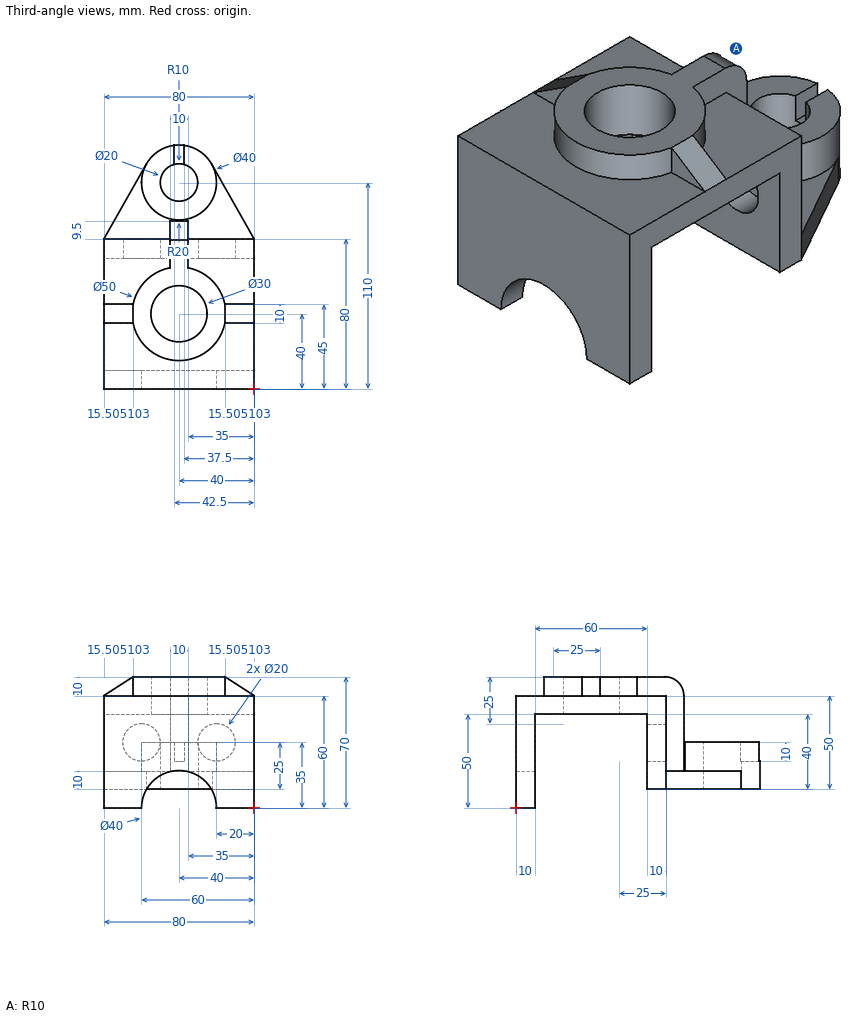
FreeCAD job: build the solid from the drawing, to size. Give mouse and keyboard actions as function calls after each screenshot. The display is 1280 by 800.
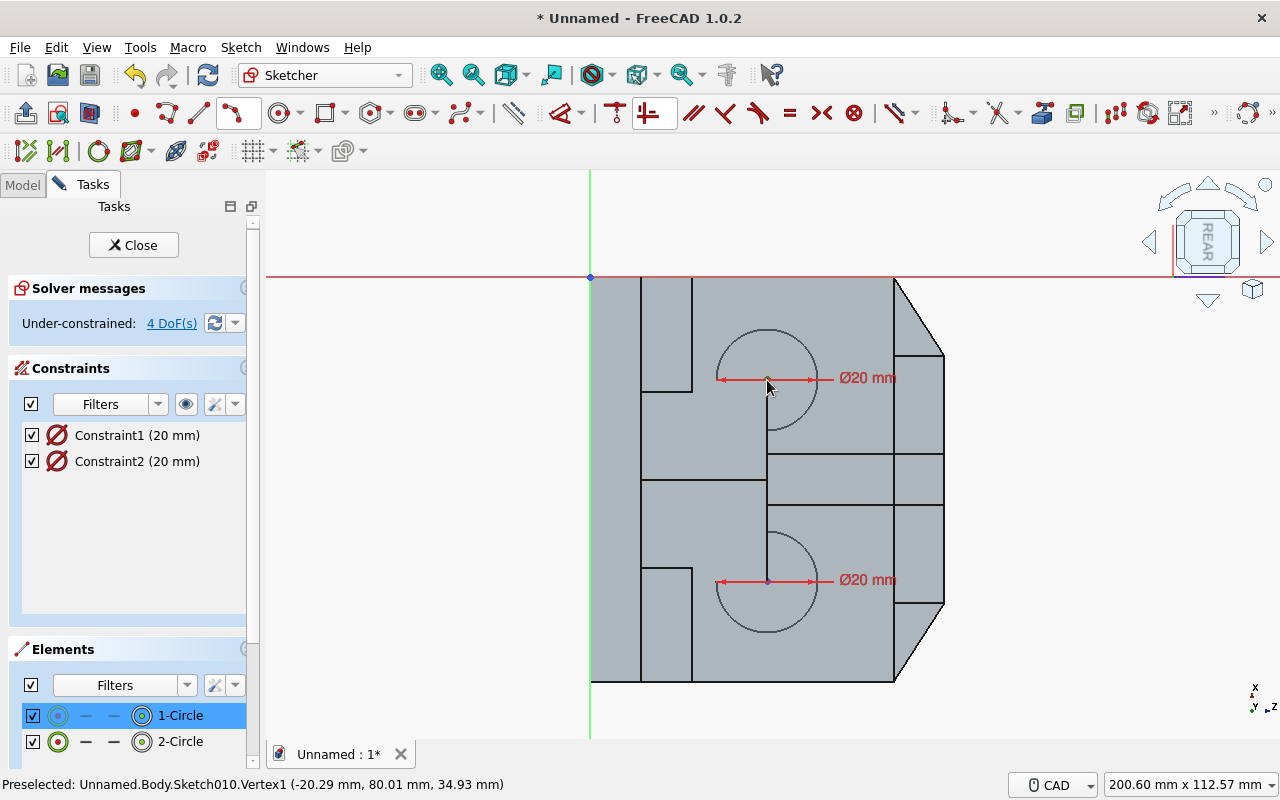
click(767, 582)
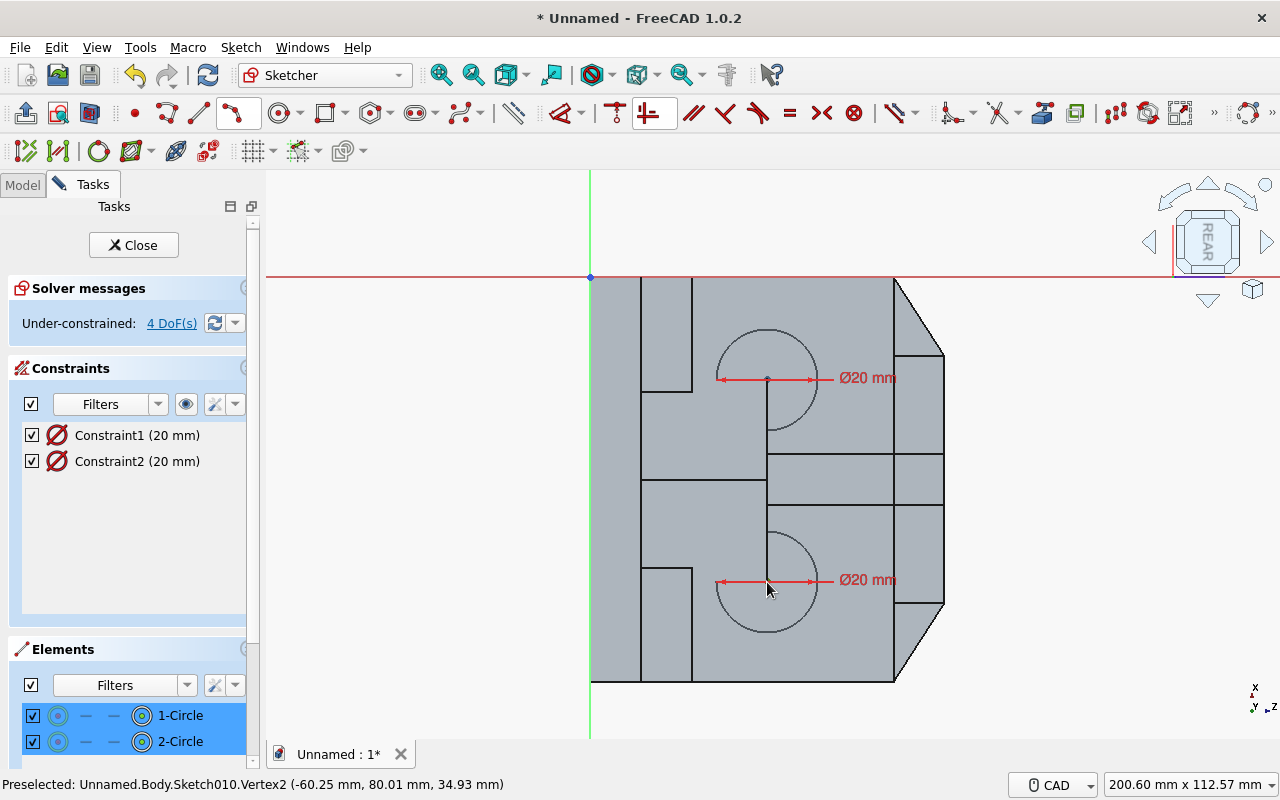
key(v)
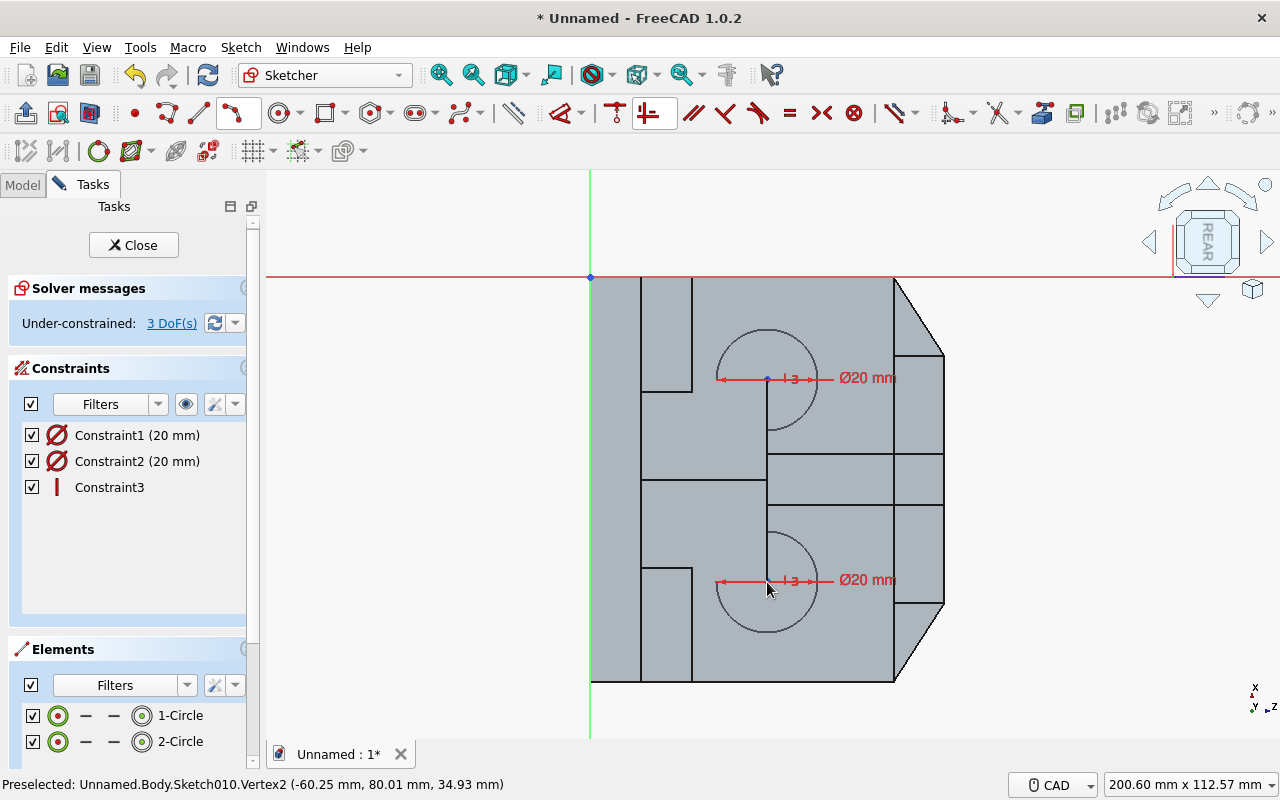
click(560, 114)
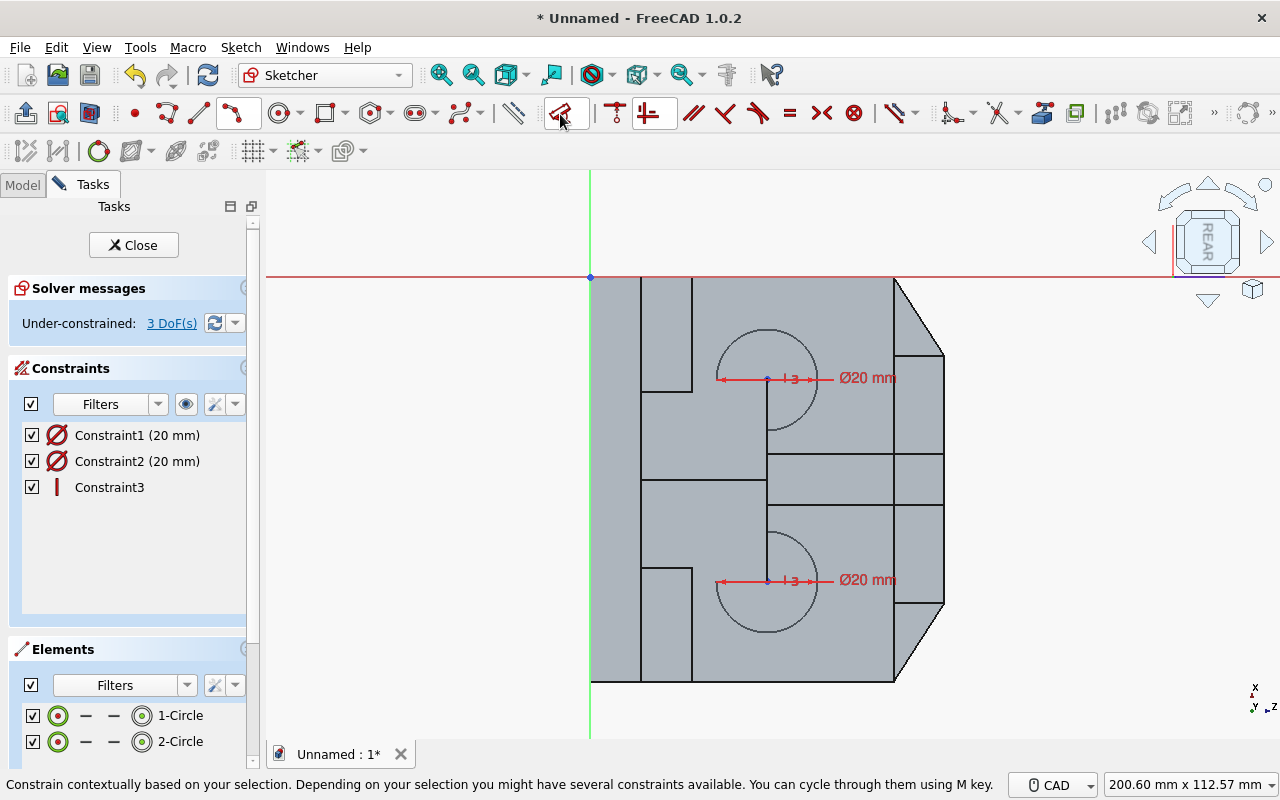
click(767, 380)
click(679, 243)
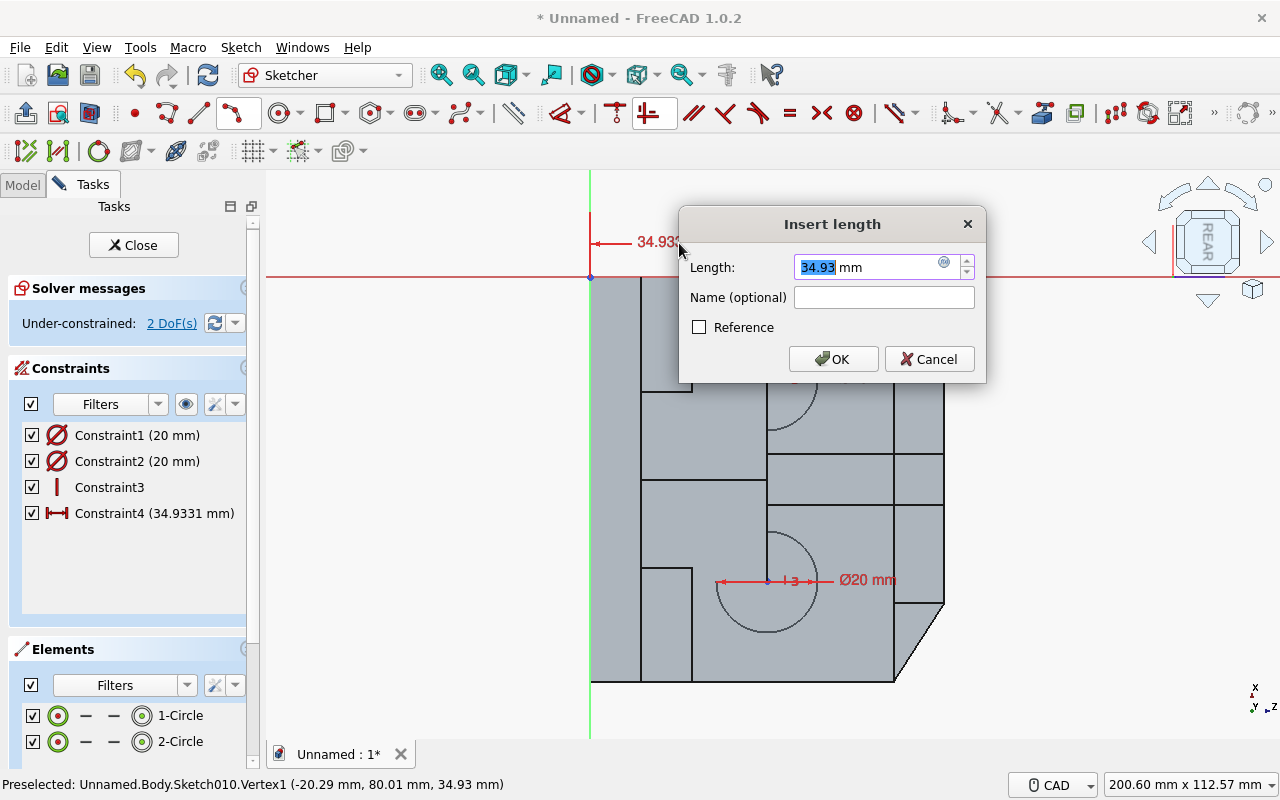
text(35)
key(Return)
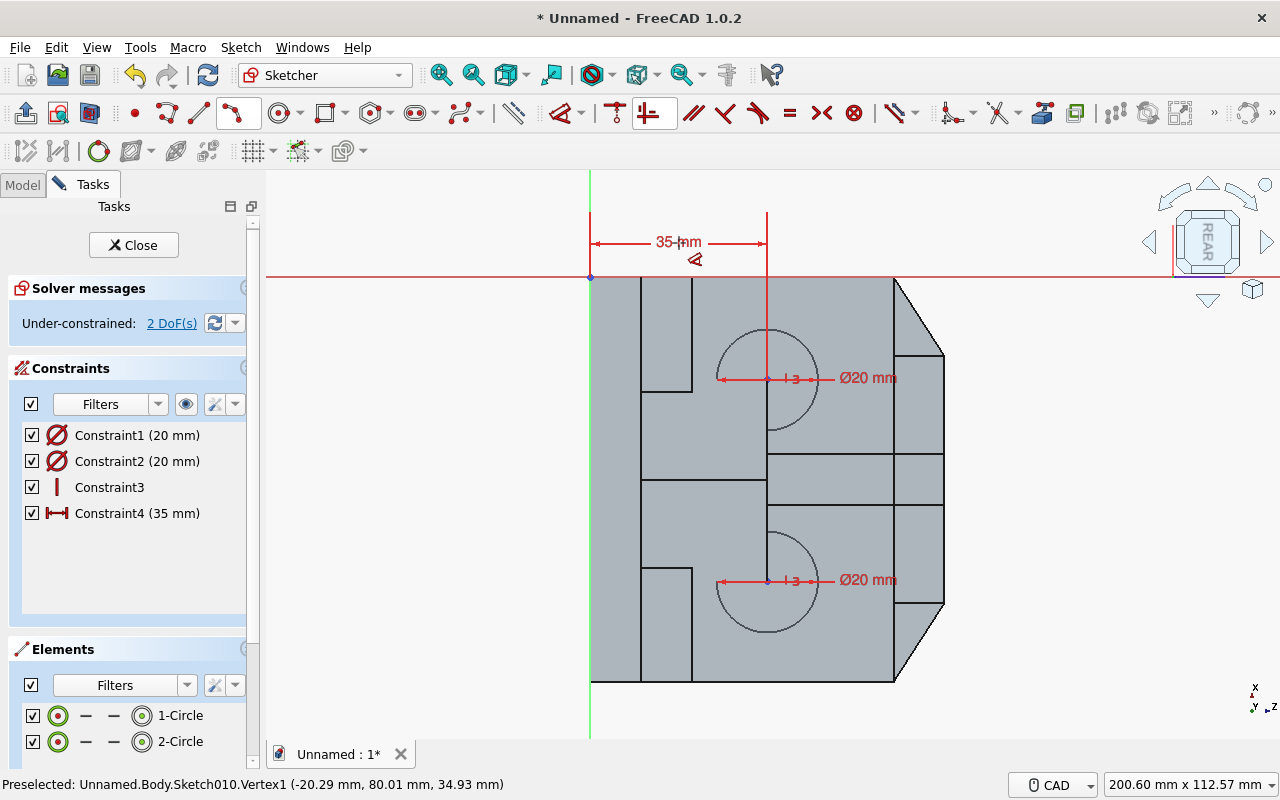
click(767, 380)
click(556, 329)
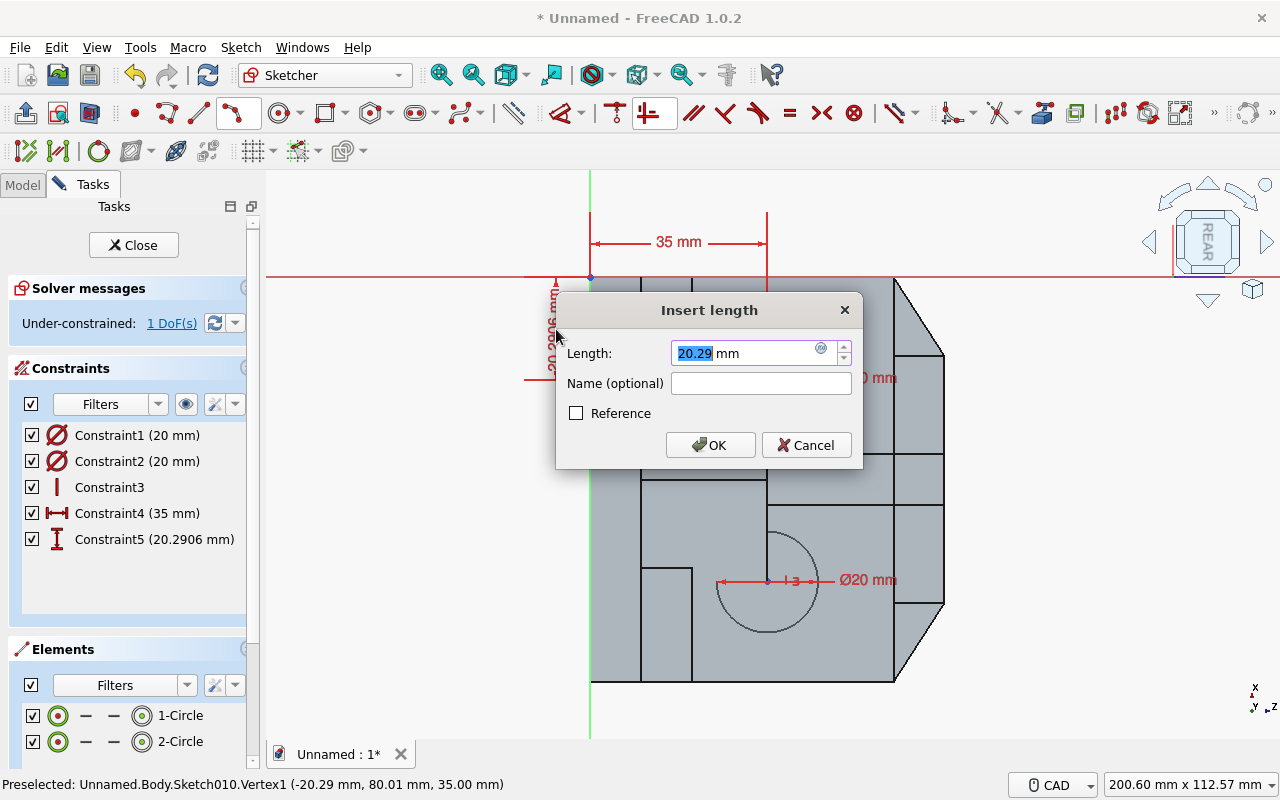
text(20)
key(Return)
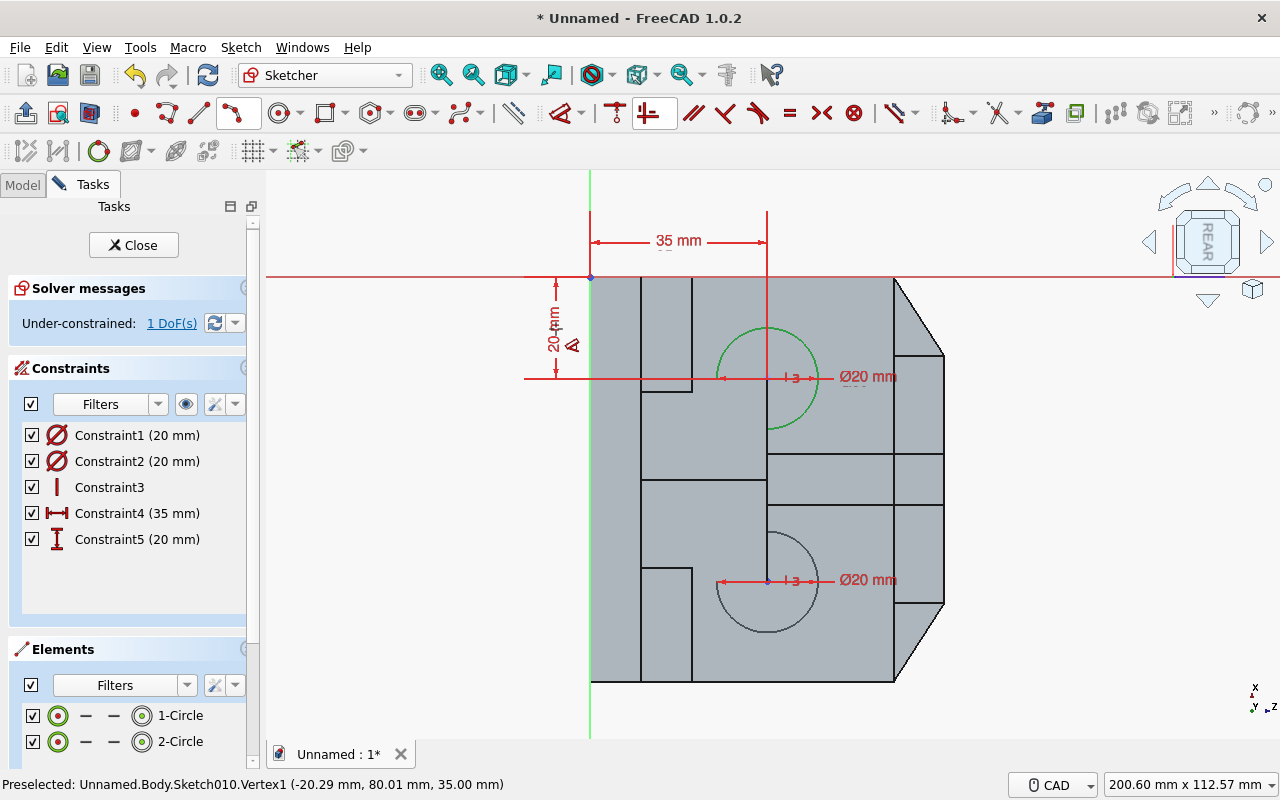
click(767, 582)
click(556, 430)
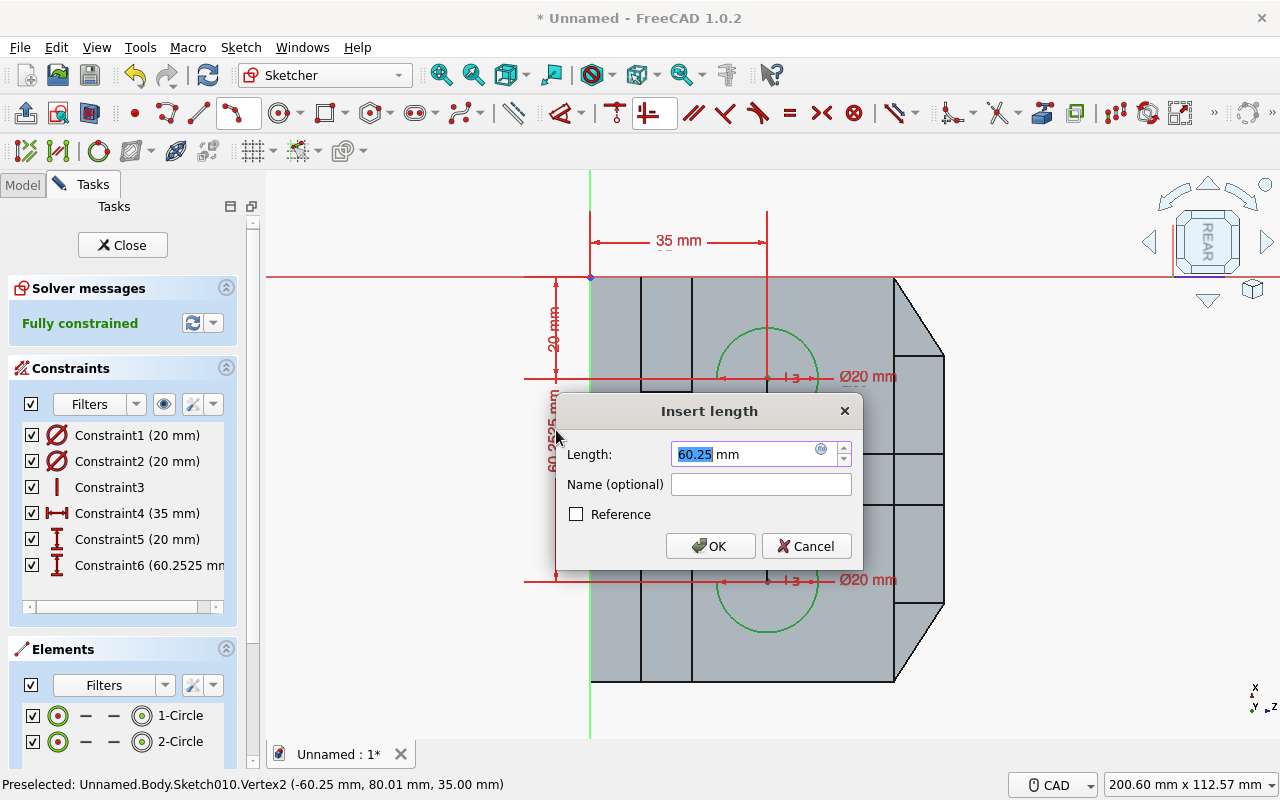
text(60)
key(Return)
key(Escape)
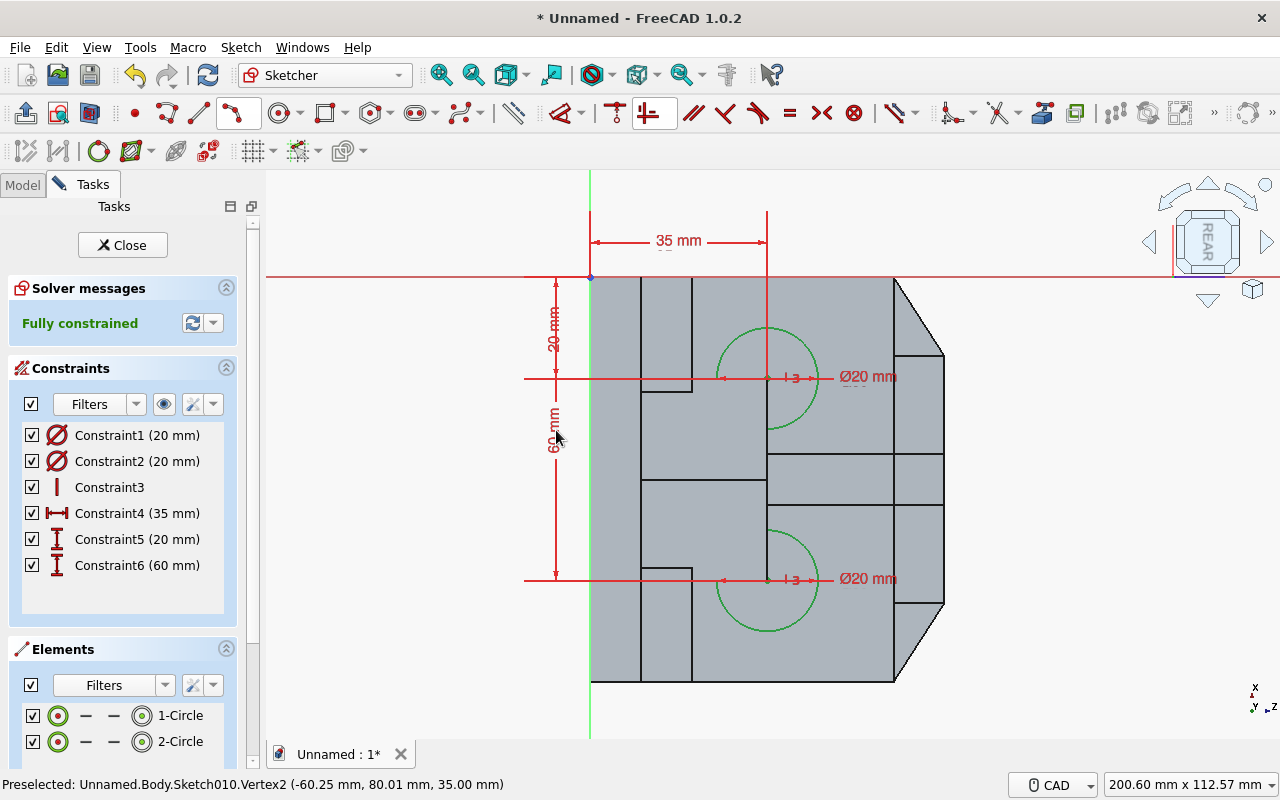
click(123, 245)